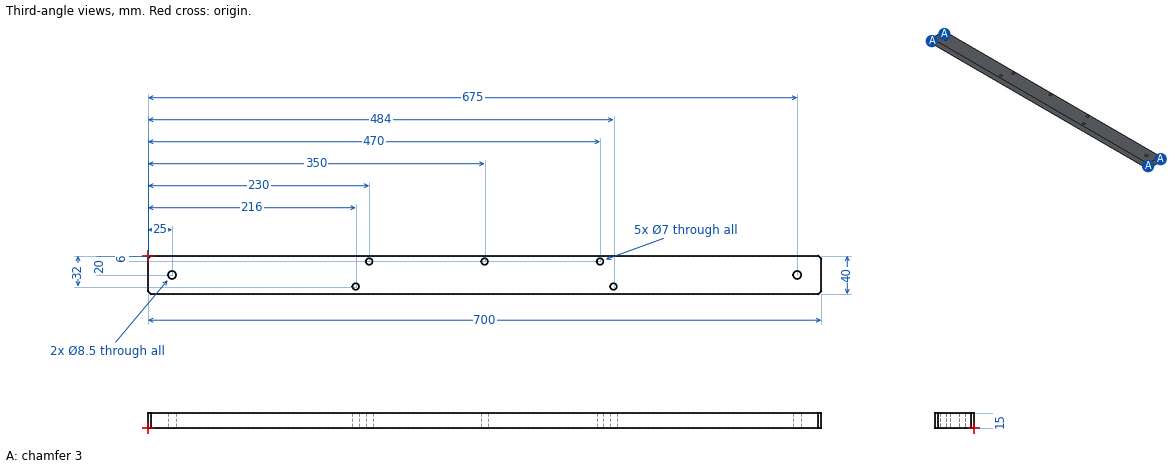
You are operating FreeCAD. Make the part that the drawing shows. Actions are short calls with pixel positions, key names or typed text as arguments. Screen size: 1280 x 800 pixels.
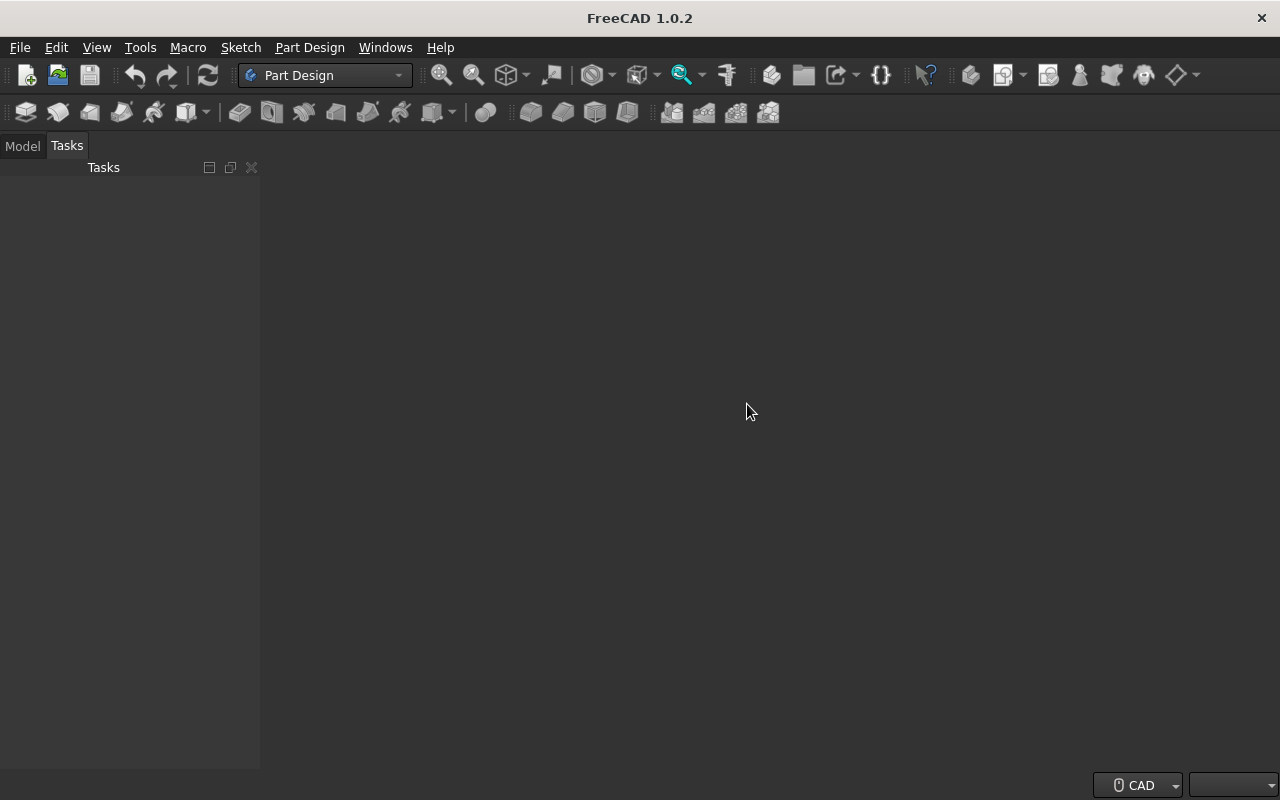
click(26, 76)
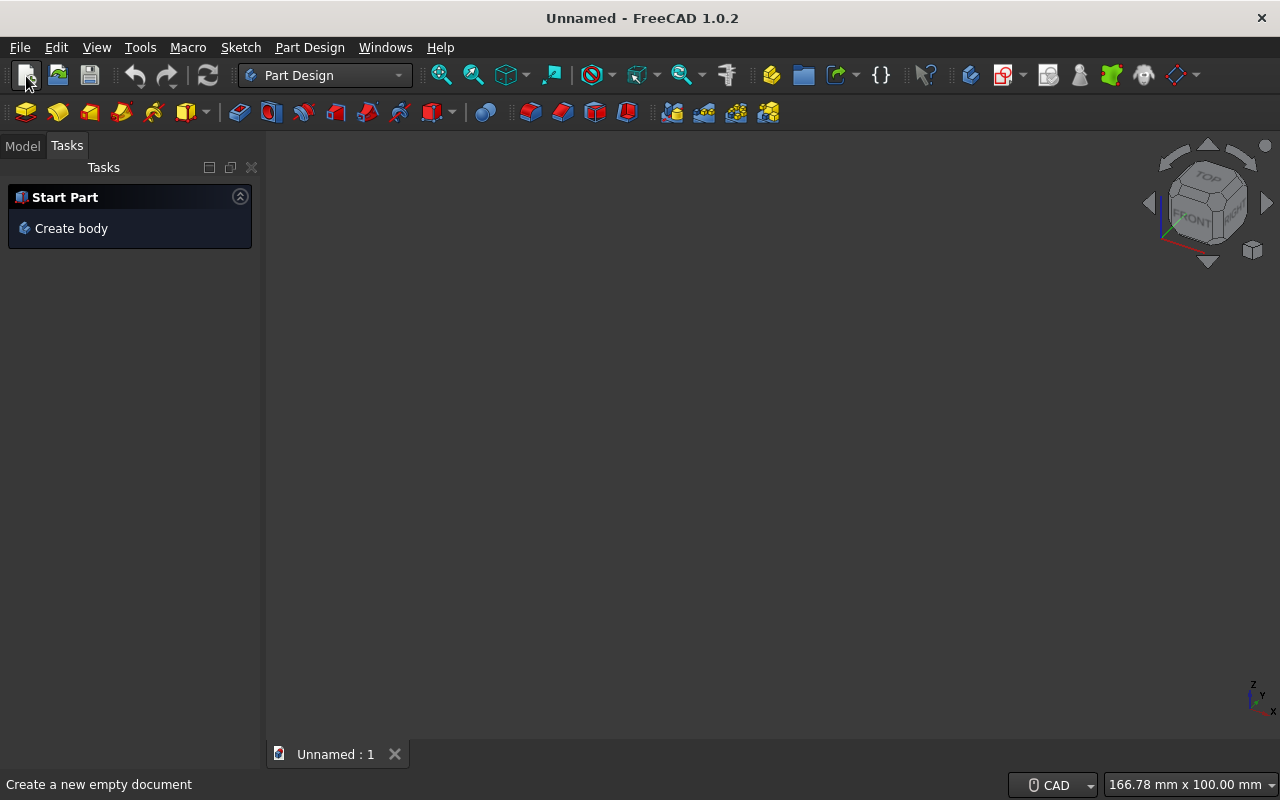
click(1004, 76)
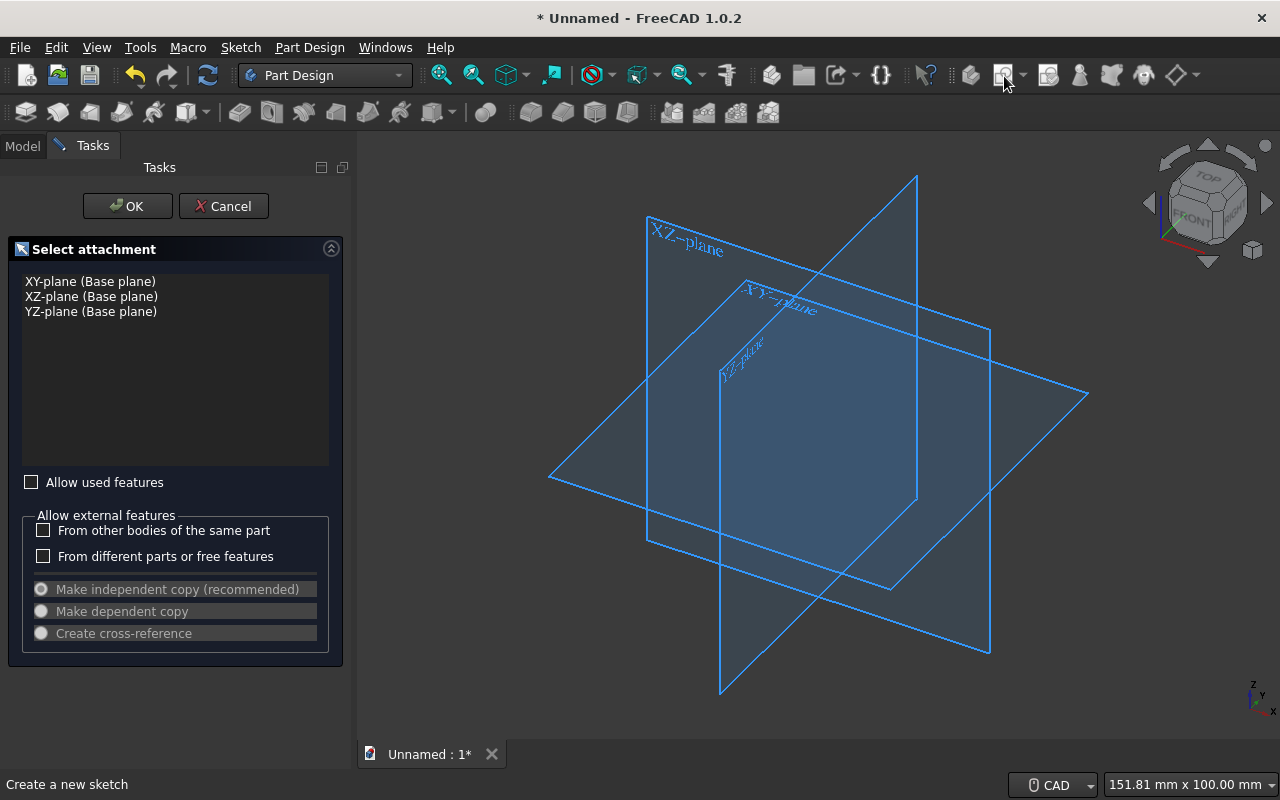
click(82, 282)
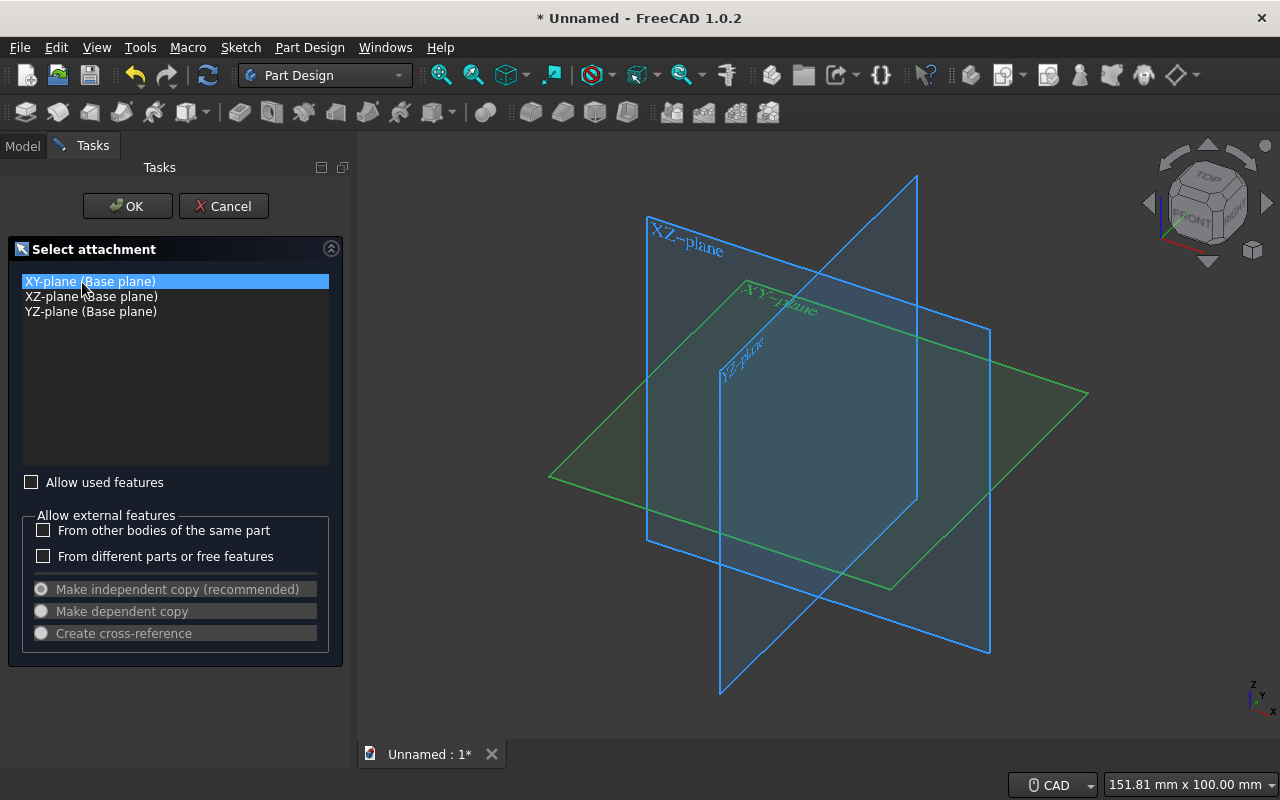
click(128, 206)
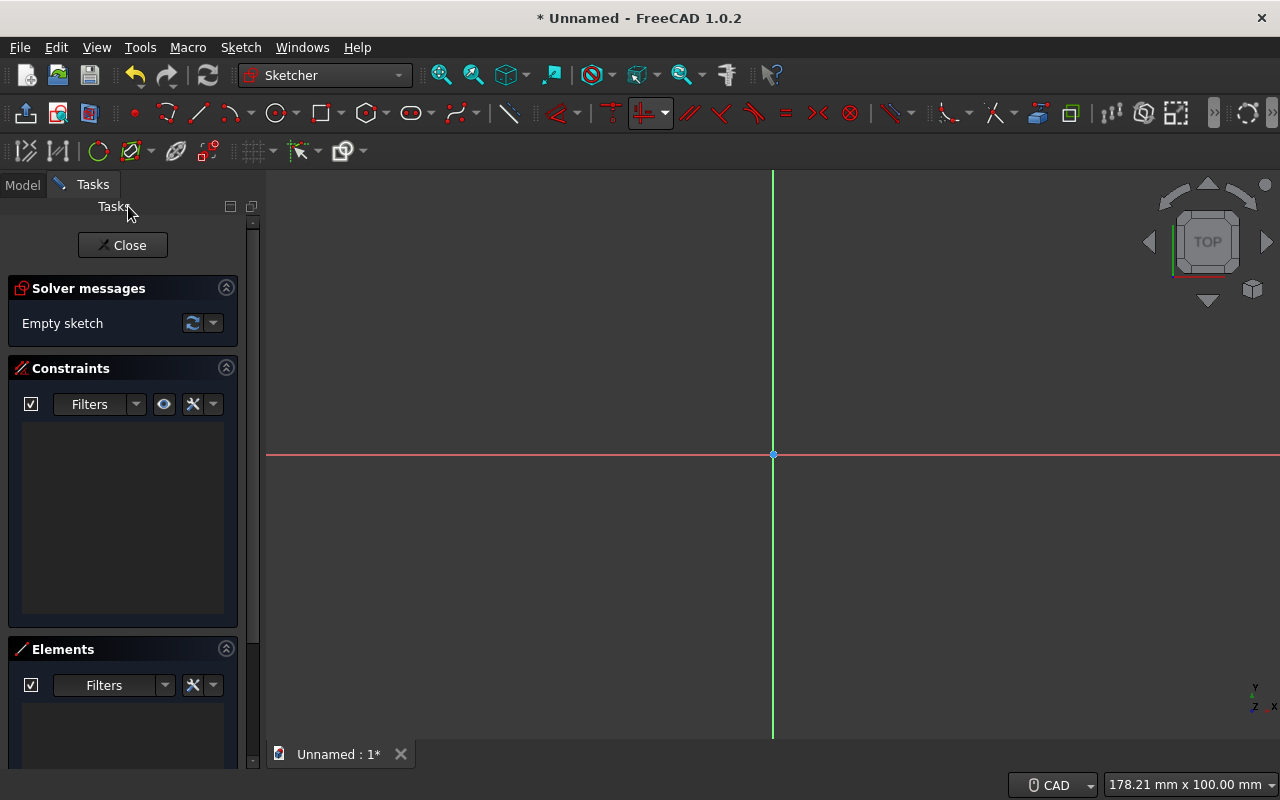
scroll(382, 437, down, 10)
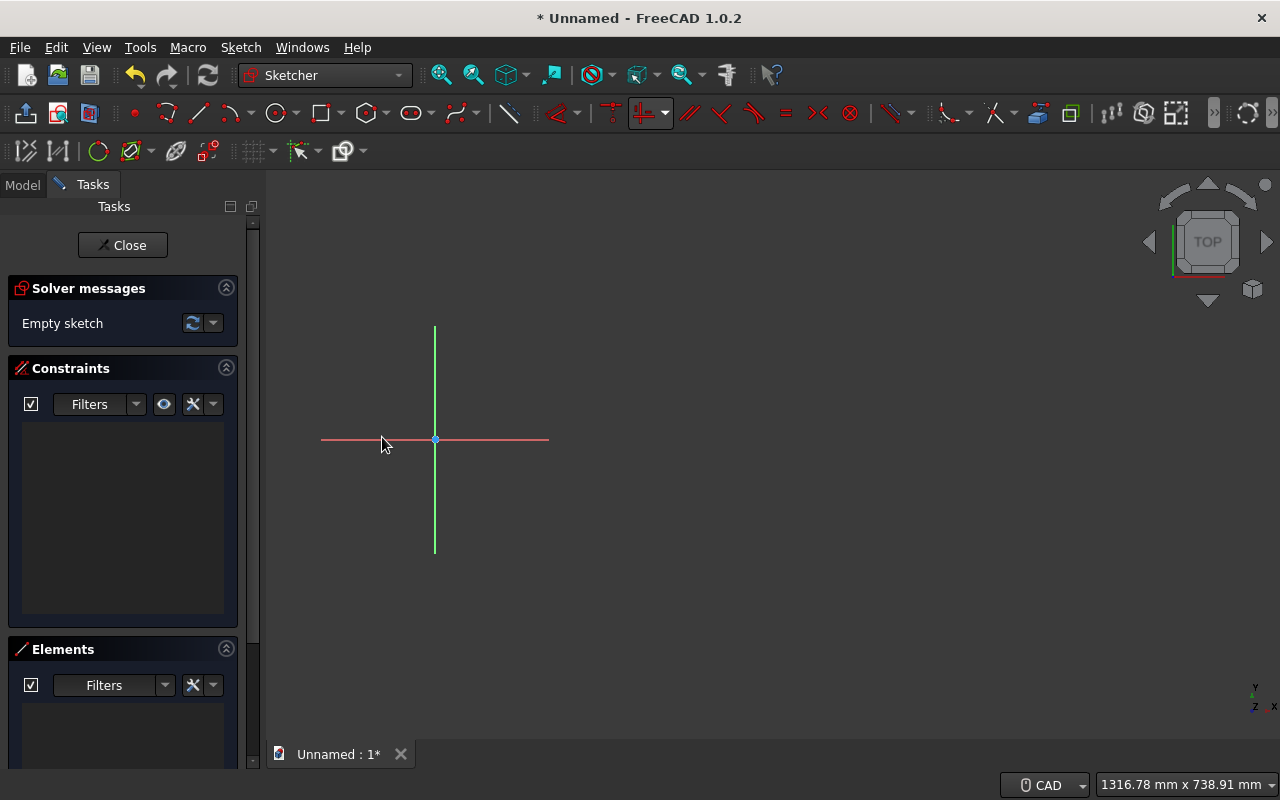
click(322, 114)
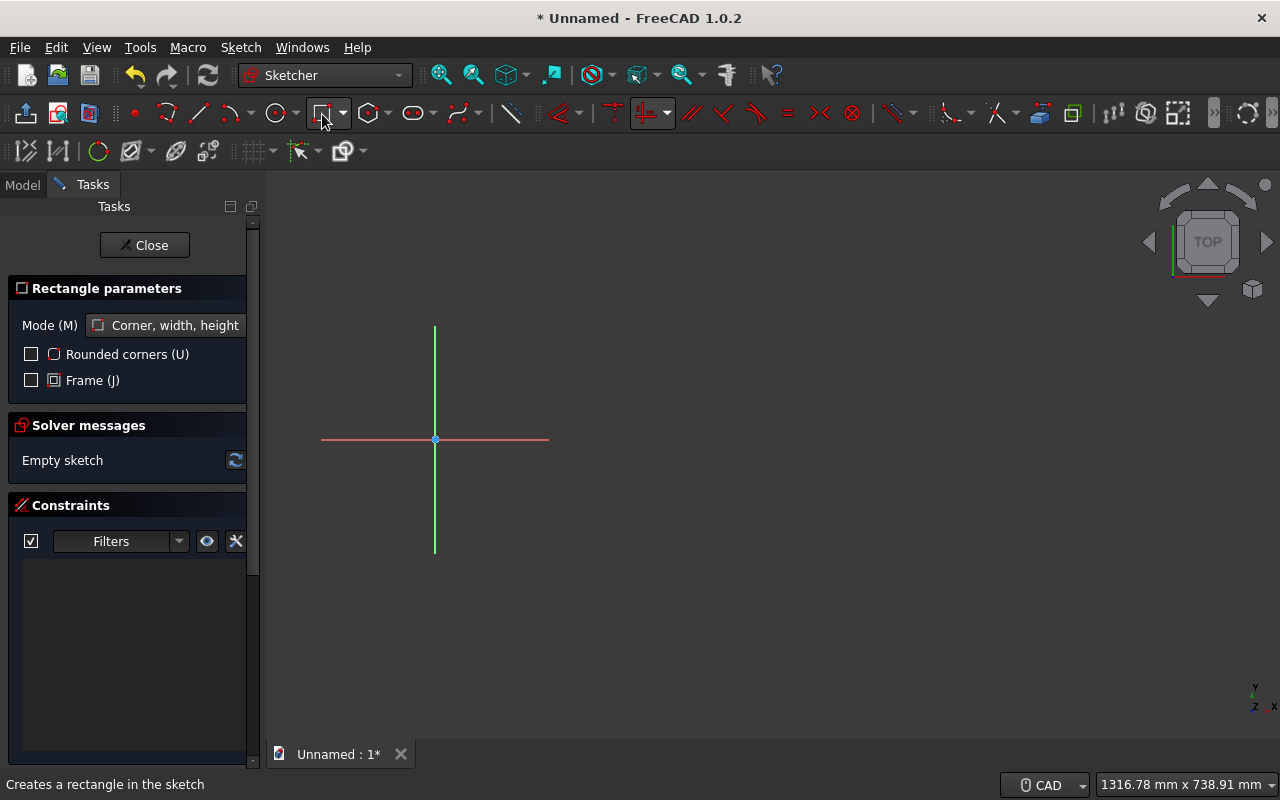
click(435, 440)
move(974, 471)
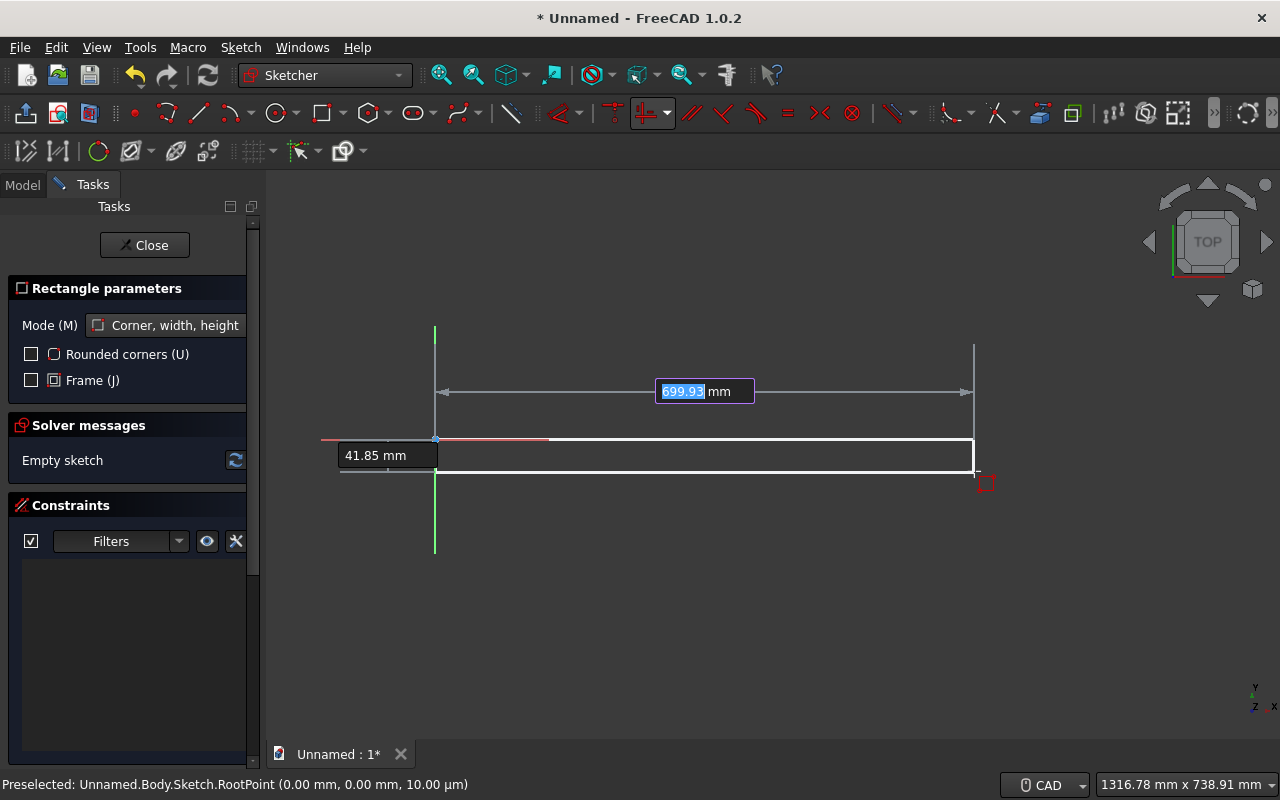
text(700)
key(Tab)
text(40)
key(Return)
key(Escape)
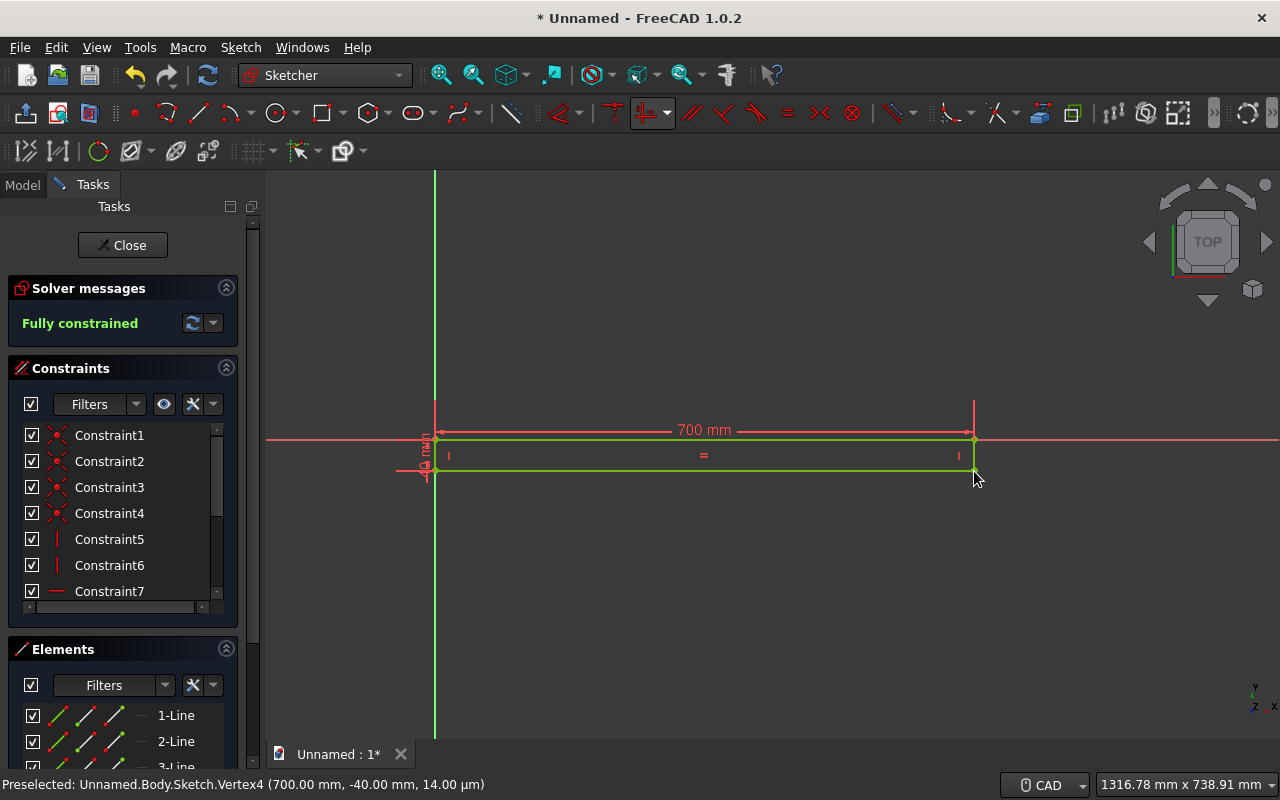
click(123, 245)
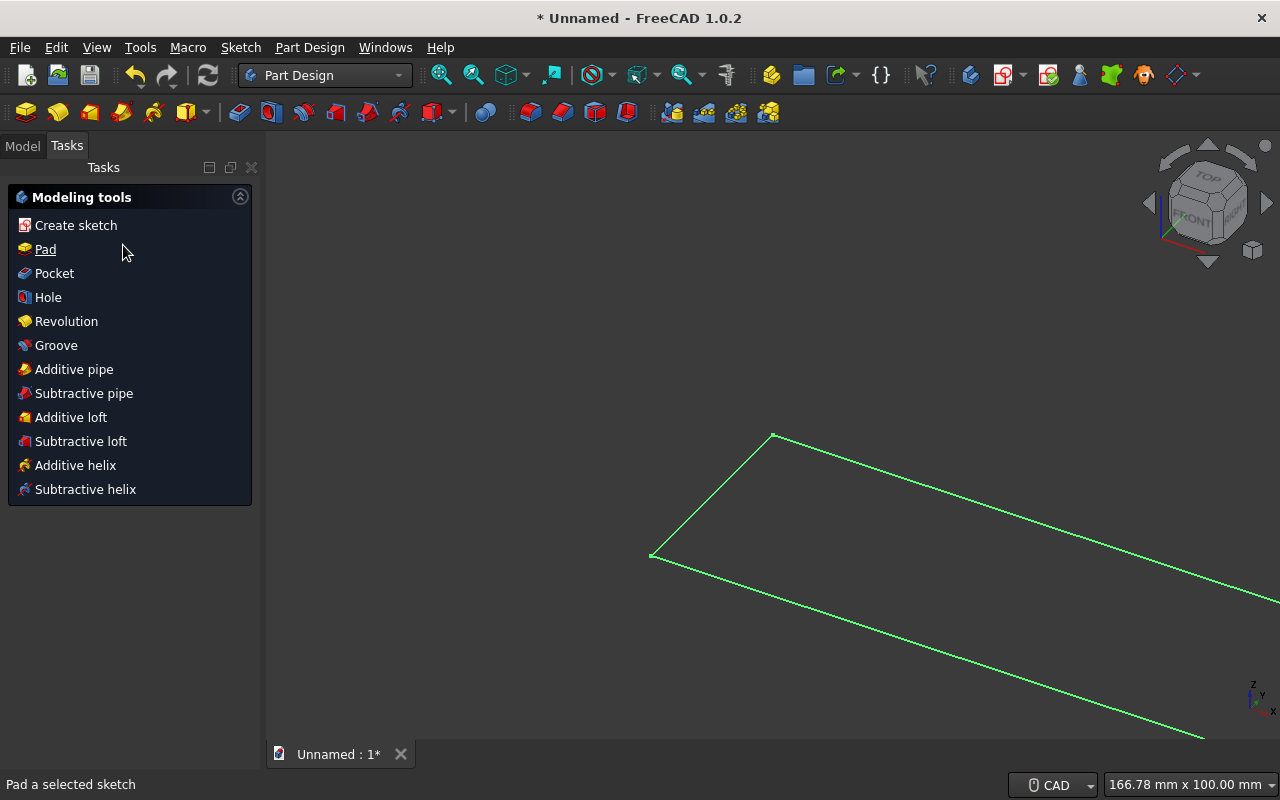
click(26, 112)